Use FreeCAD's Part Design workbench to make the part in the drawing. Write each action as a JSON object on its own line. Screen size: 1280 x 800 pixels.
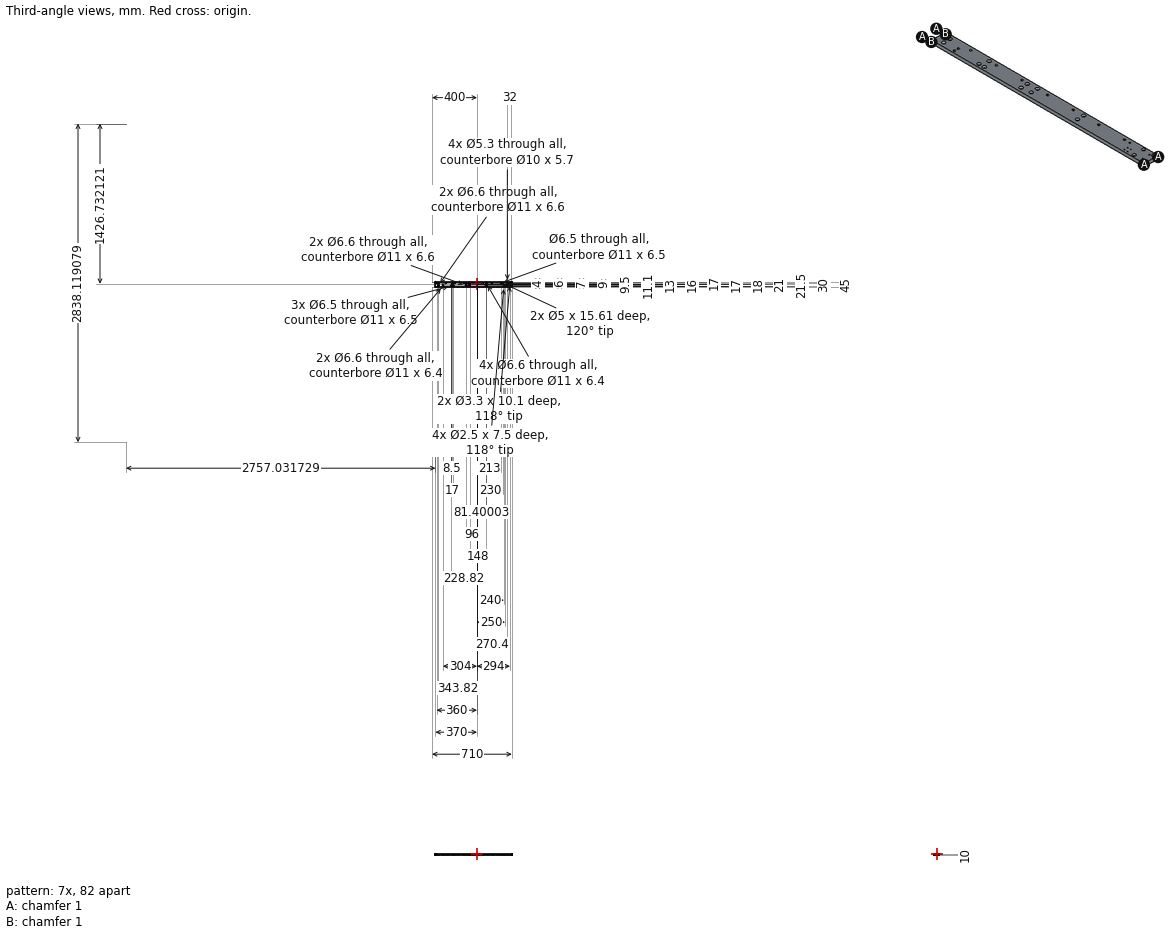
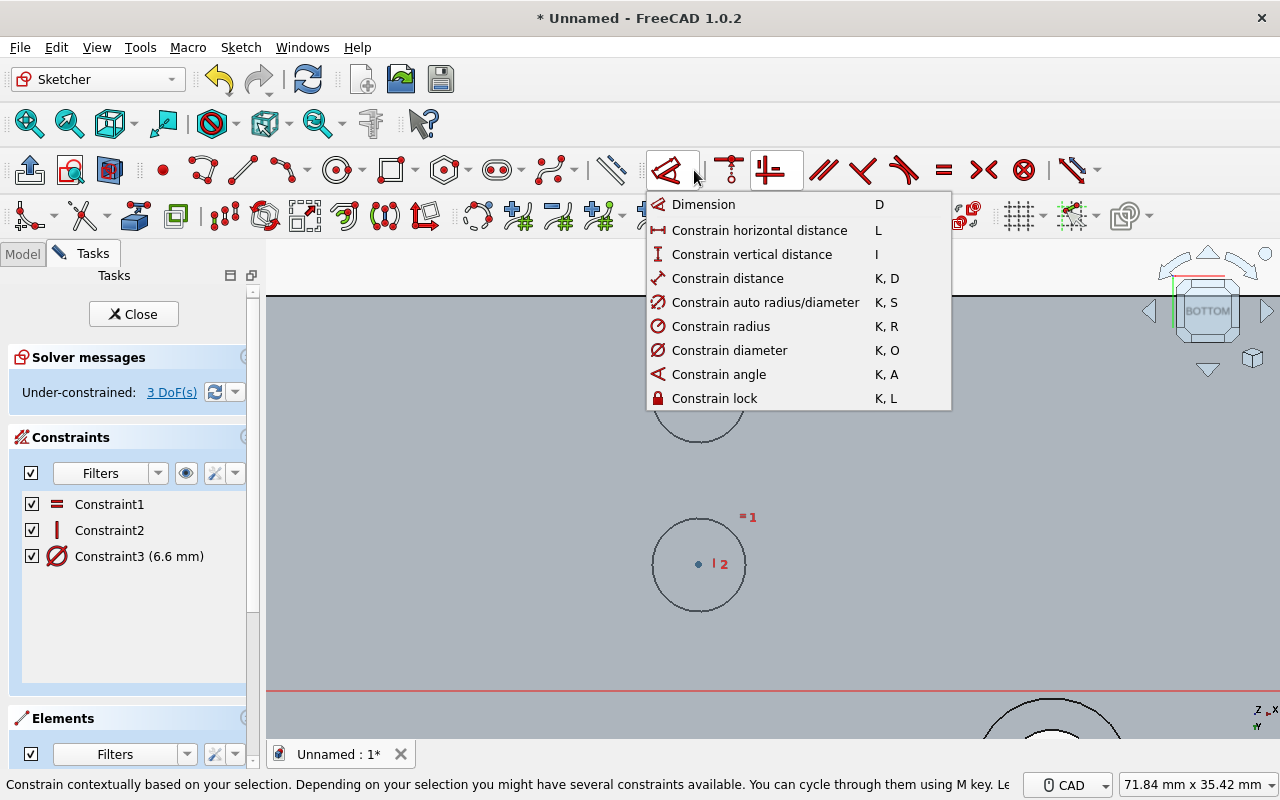
{"action": "left_click", "coordinate": [799, 254]}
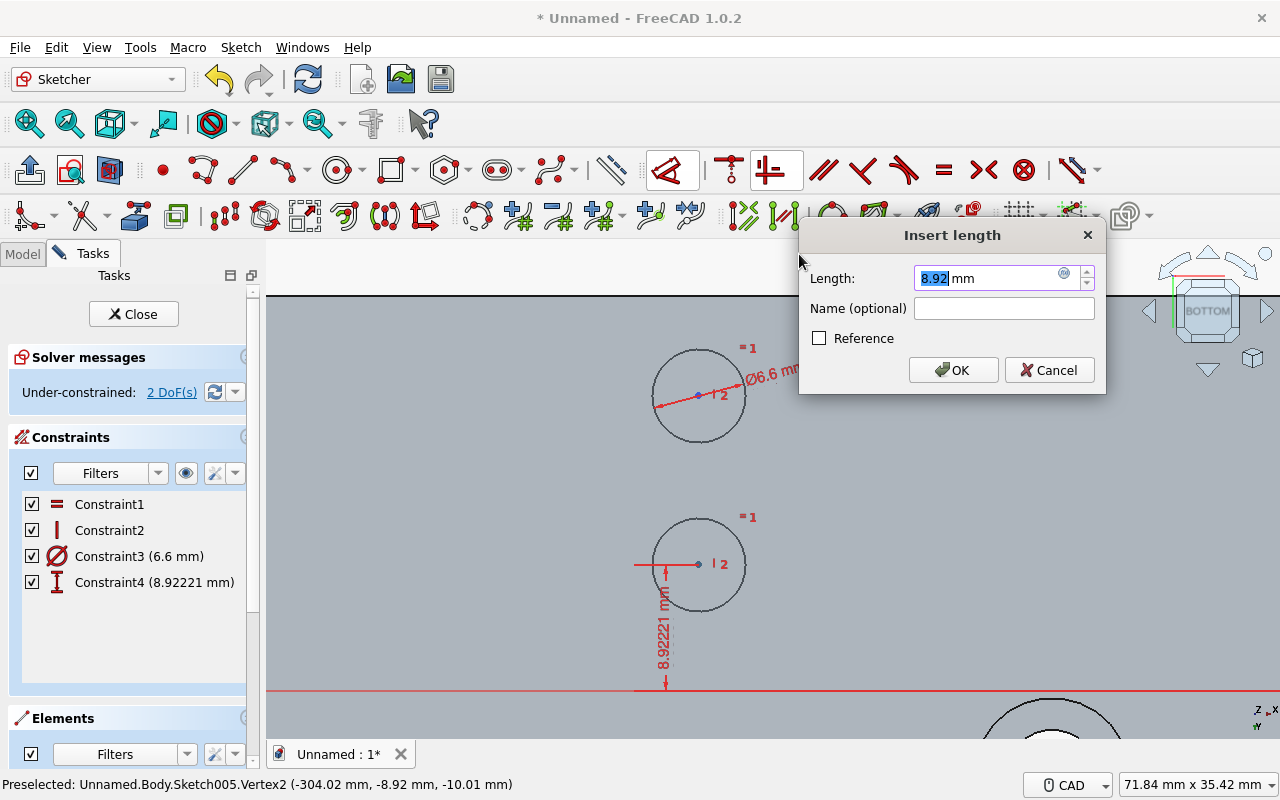
{"action": "type", "text": "9"}
{"action": "key", "text": "Return"}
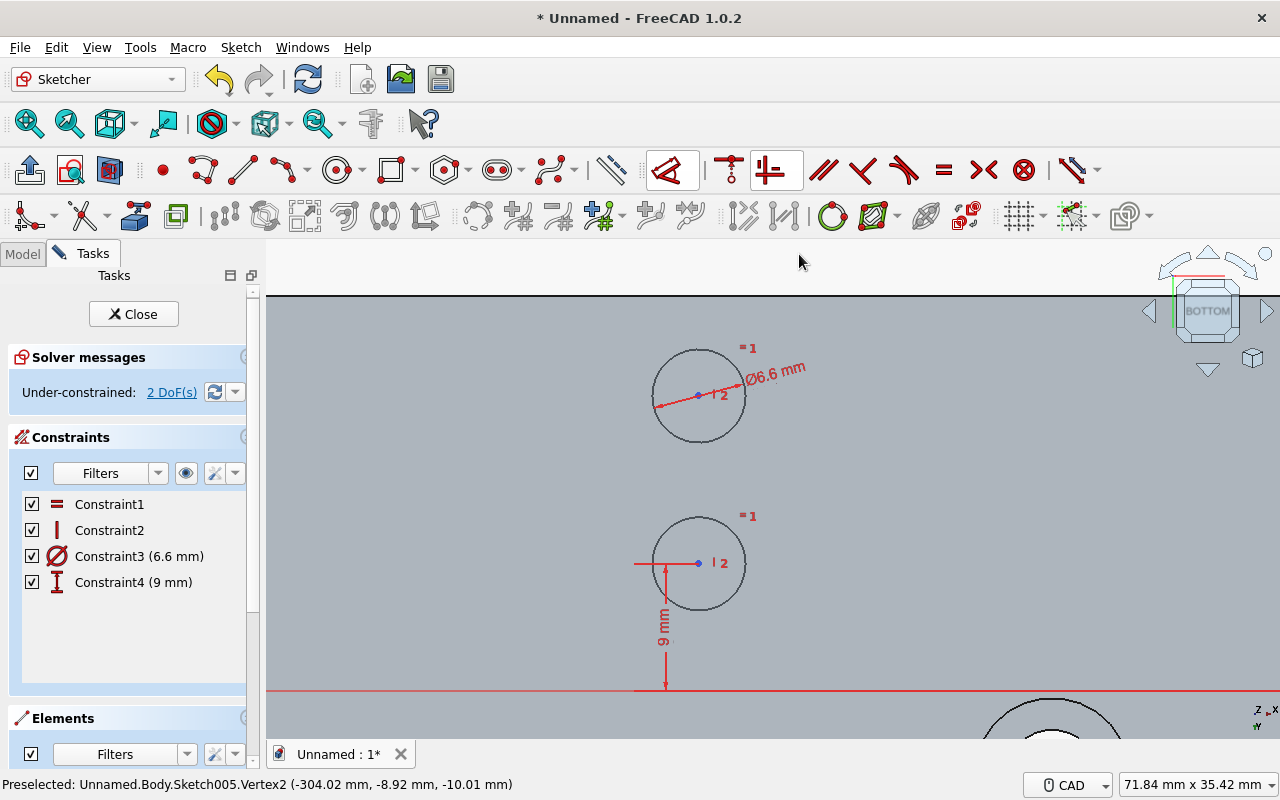
{"action": "left_click", "coordinate": [699, 396]}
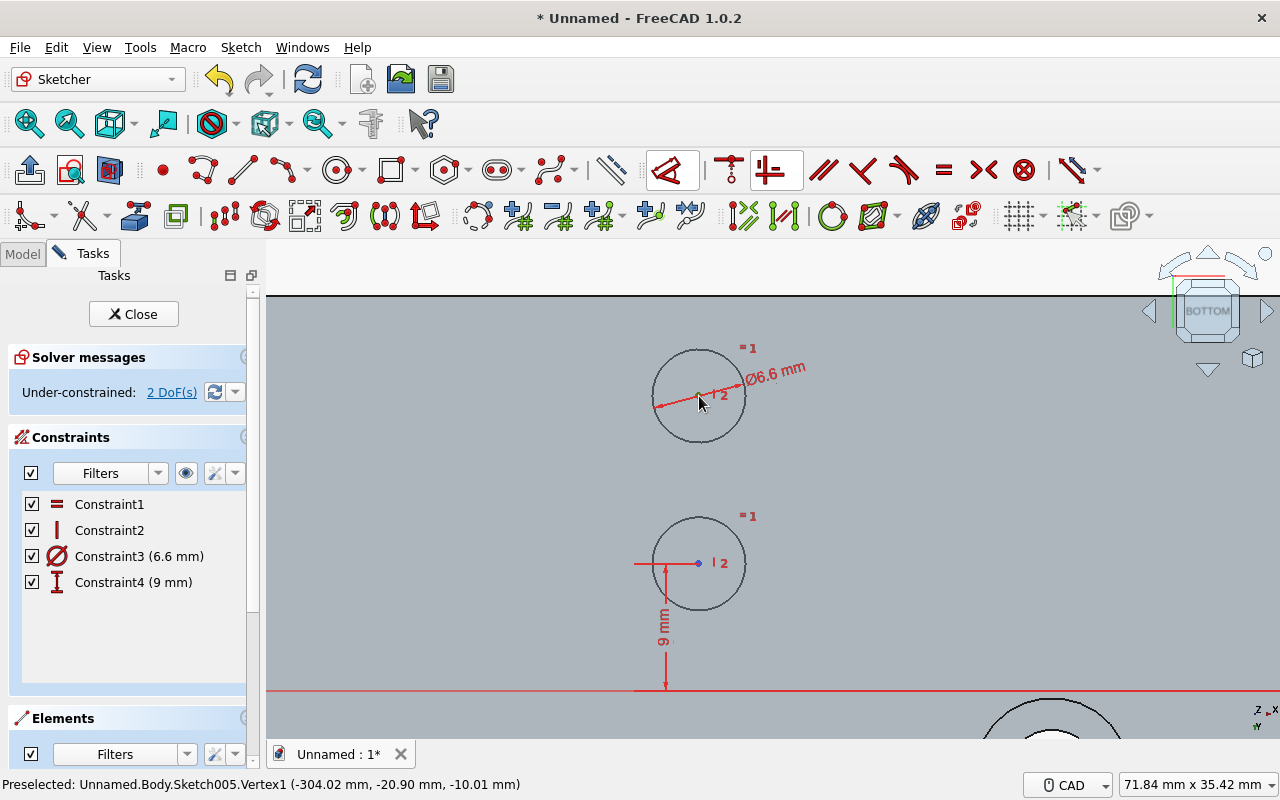
{"action": "left_click", "coordinate": [694, 170]}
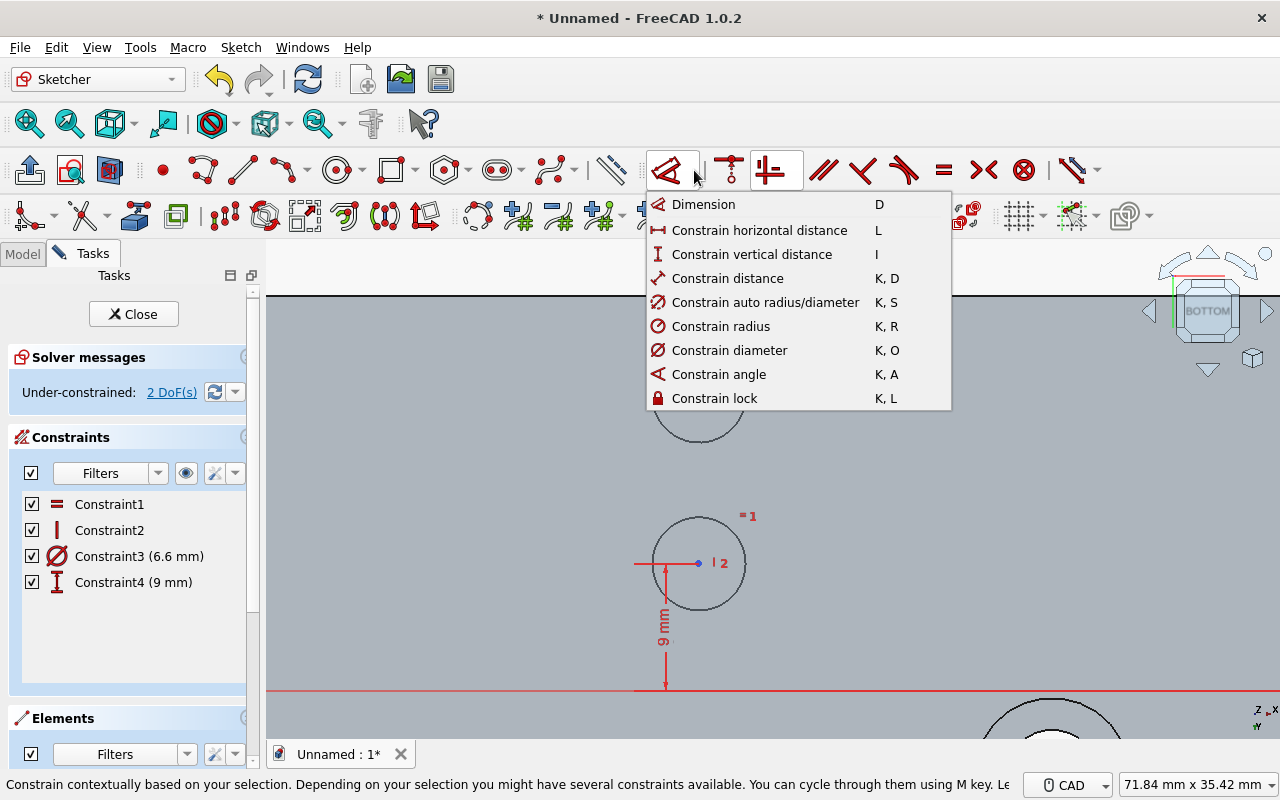
{"action": "left_click", "coordinate": [799, 254]}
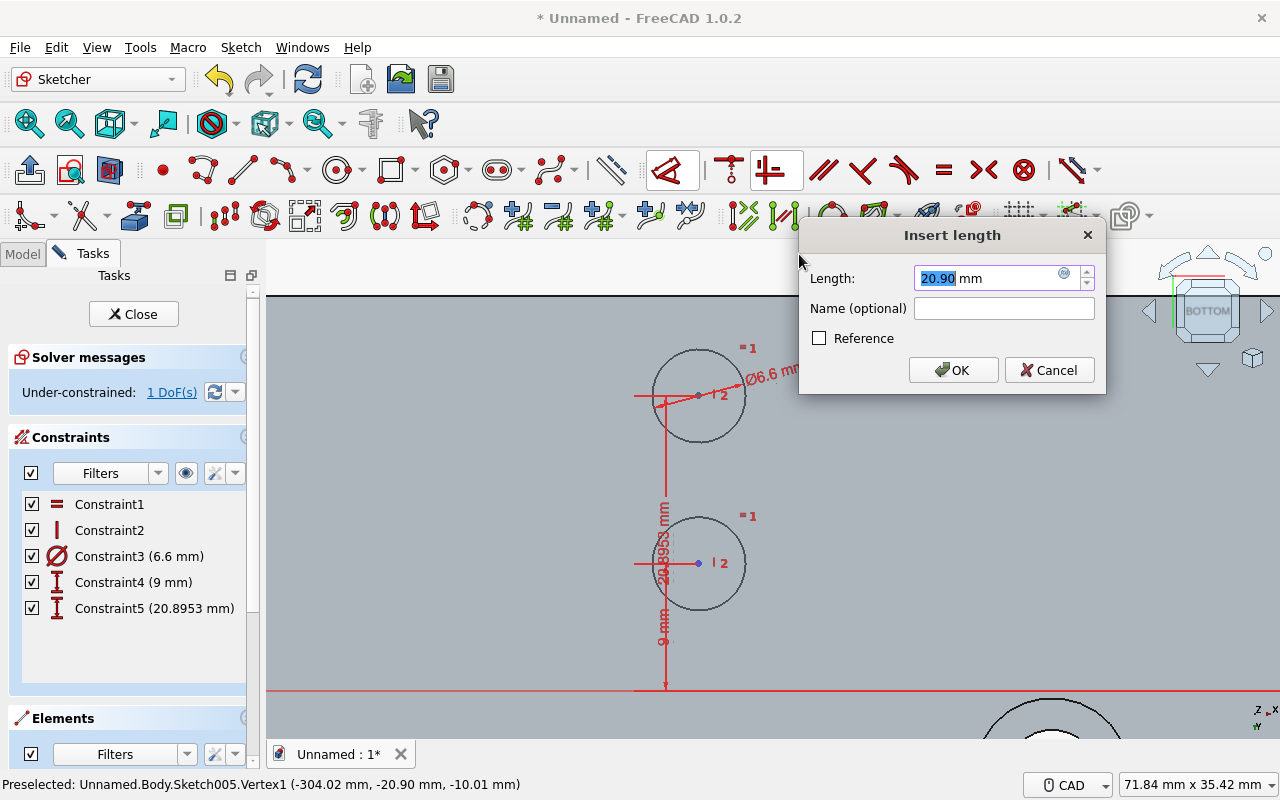
{"action": "type", "text": "21"}
{"action": "key", "text": "Return"}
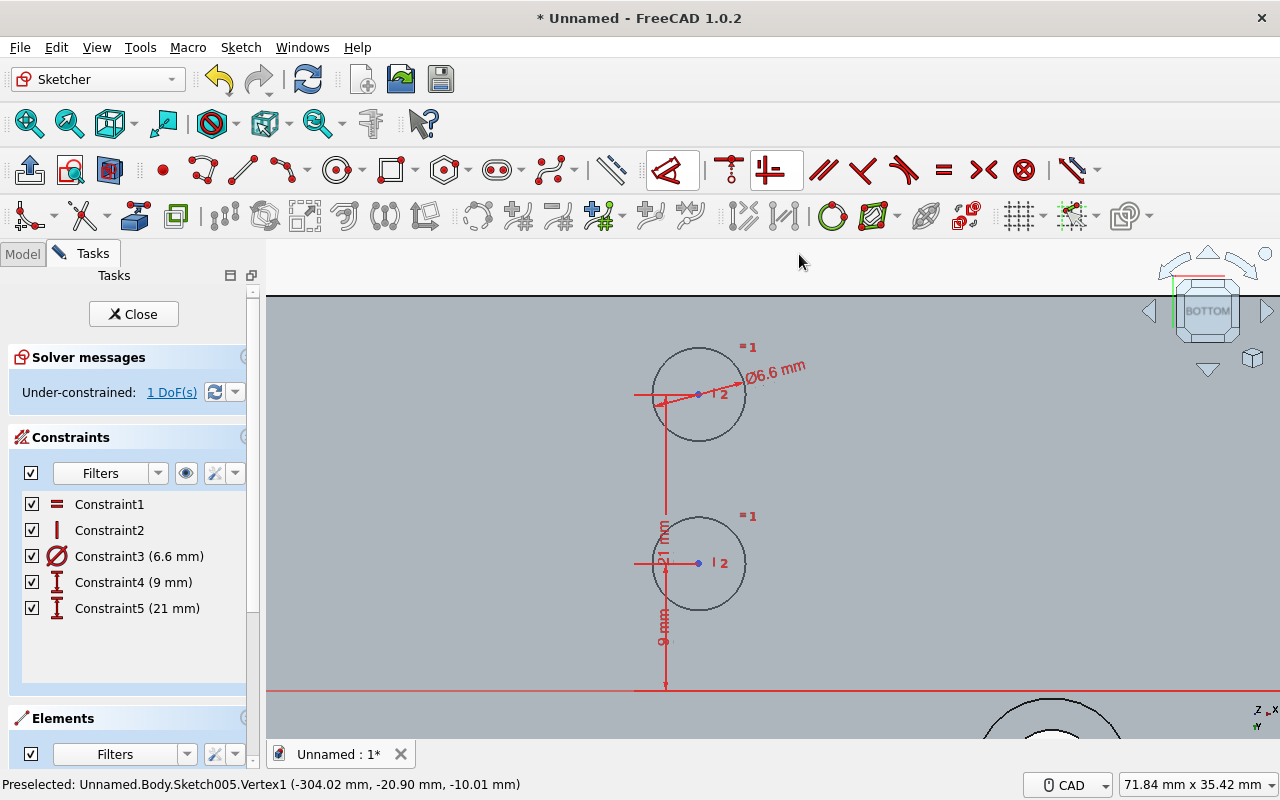
{"action": "left_click", "coordinate": [699, 395]}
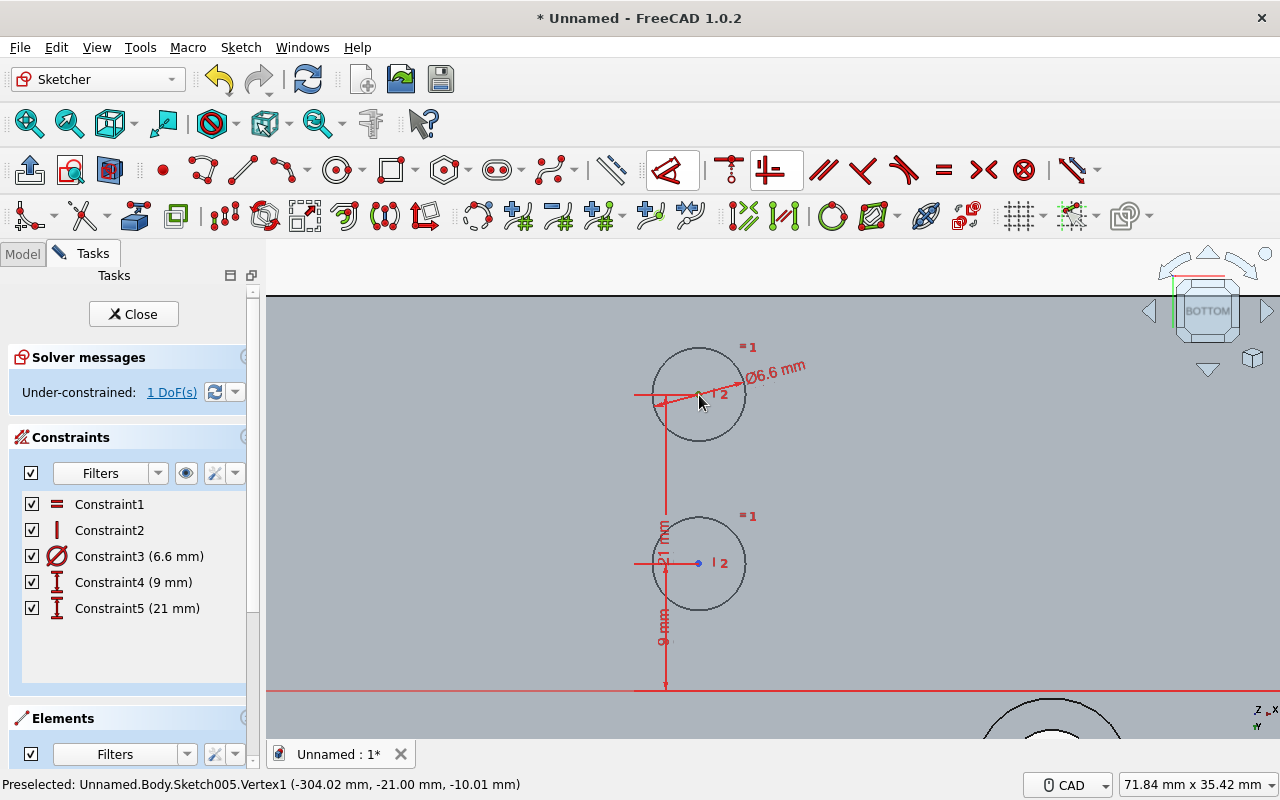
{"action": "key", "text": "l"}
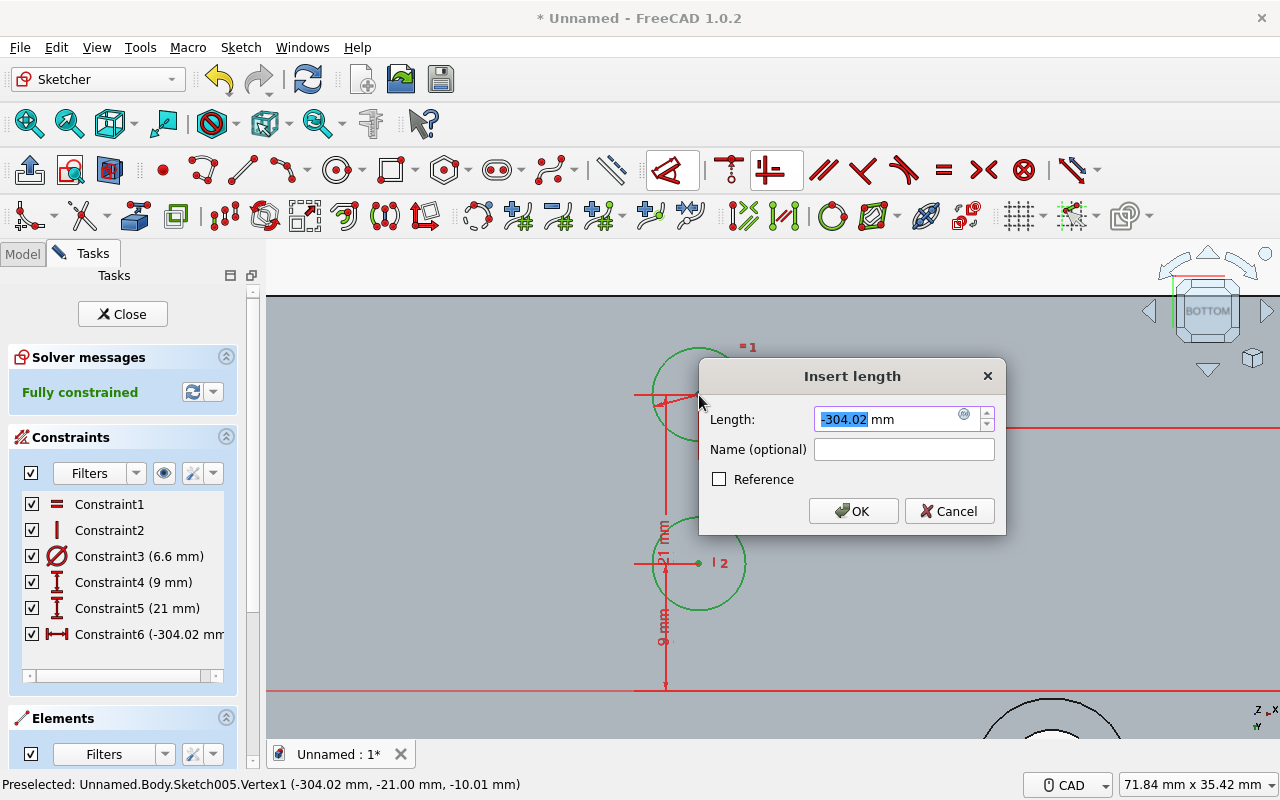
{"action": "type", "text": "-304"}
{"action": "key", "text": "Return"}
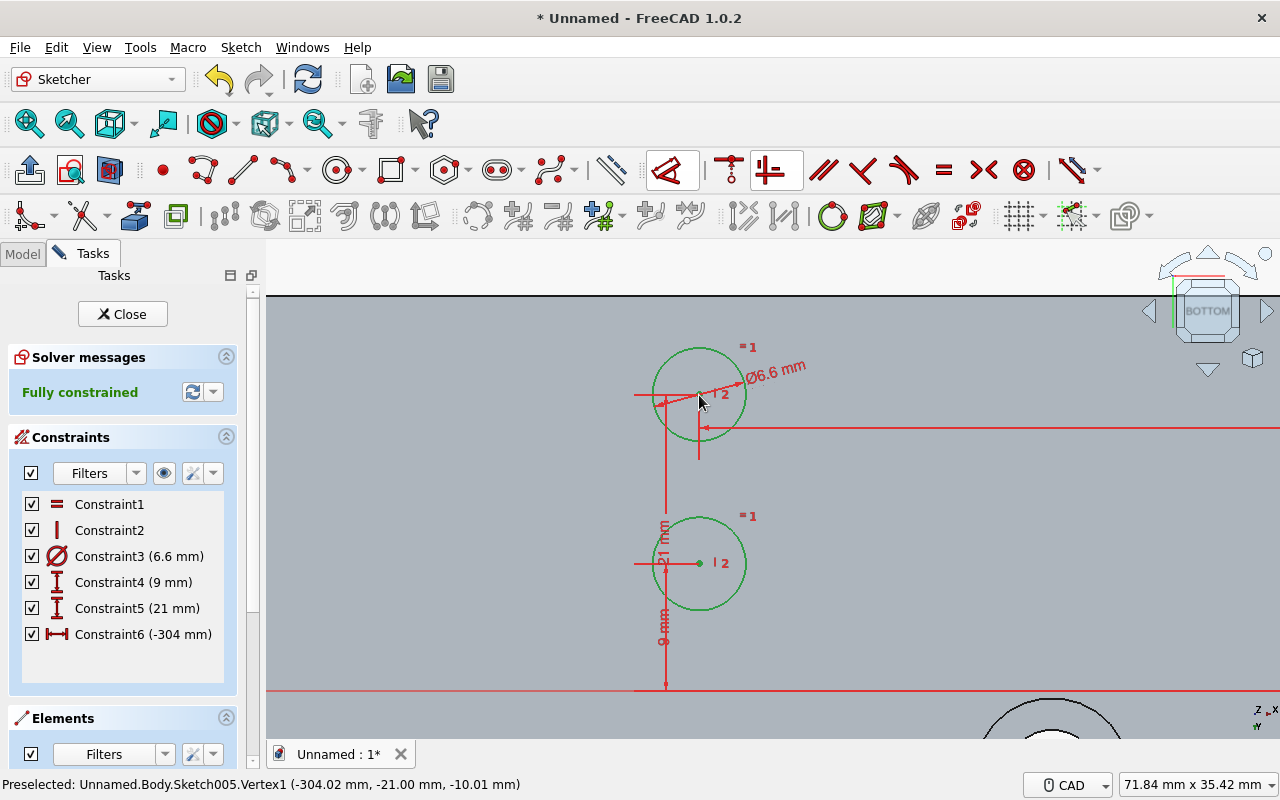
{"action": "left_click", "coordinate": [123, 314]}